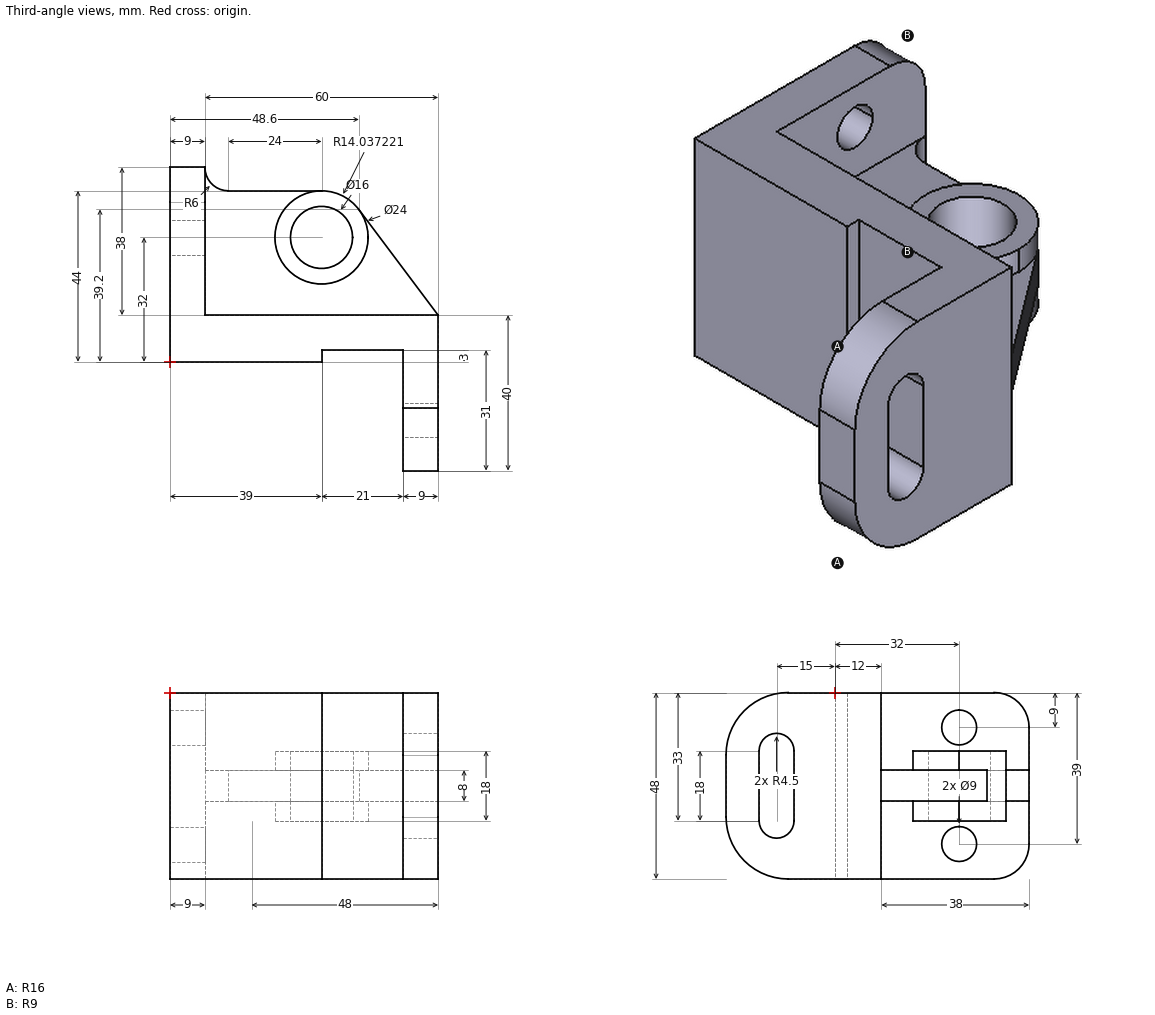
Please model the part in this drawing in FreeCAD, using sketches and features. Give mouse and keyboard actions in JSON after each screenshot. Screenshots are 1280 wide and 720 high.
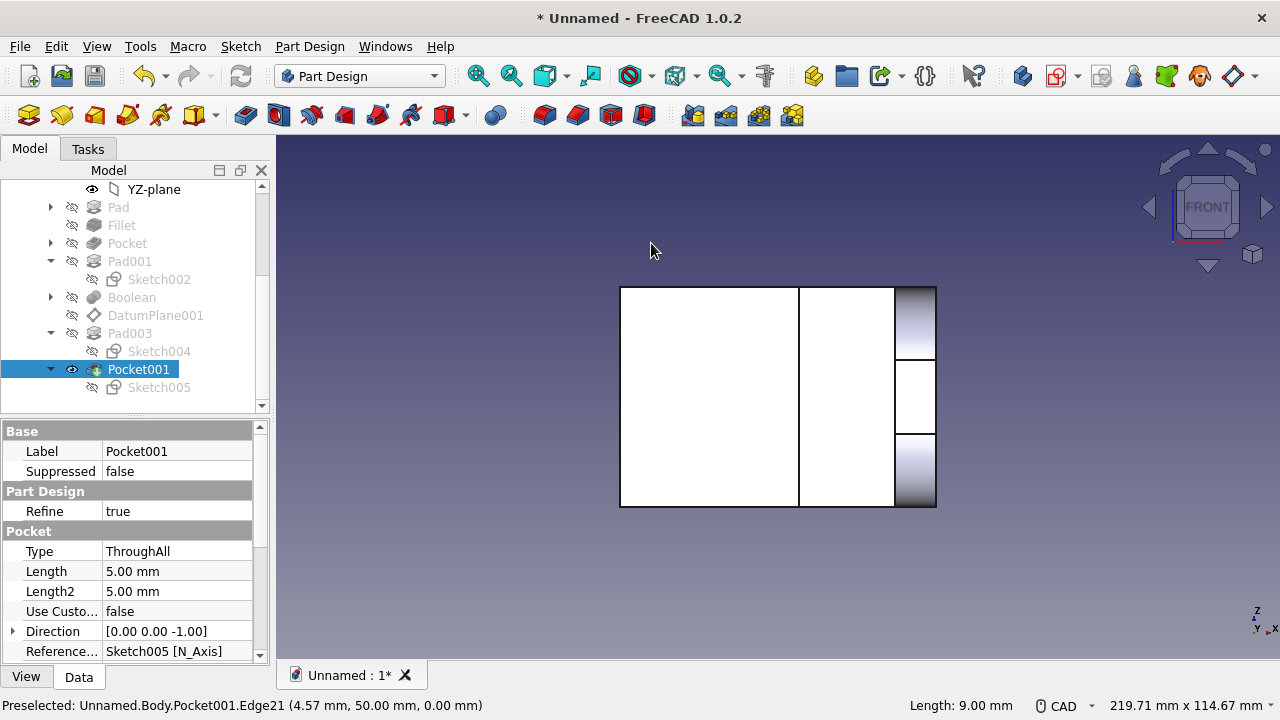
{"action": "key", "text": "3"}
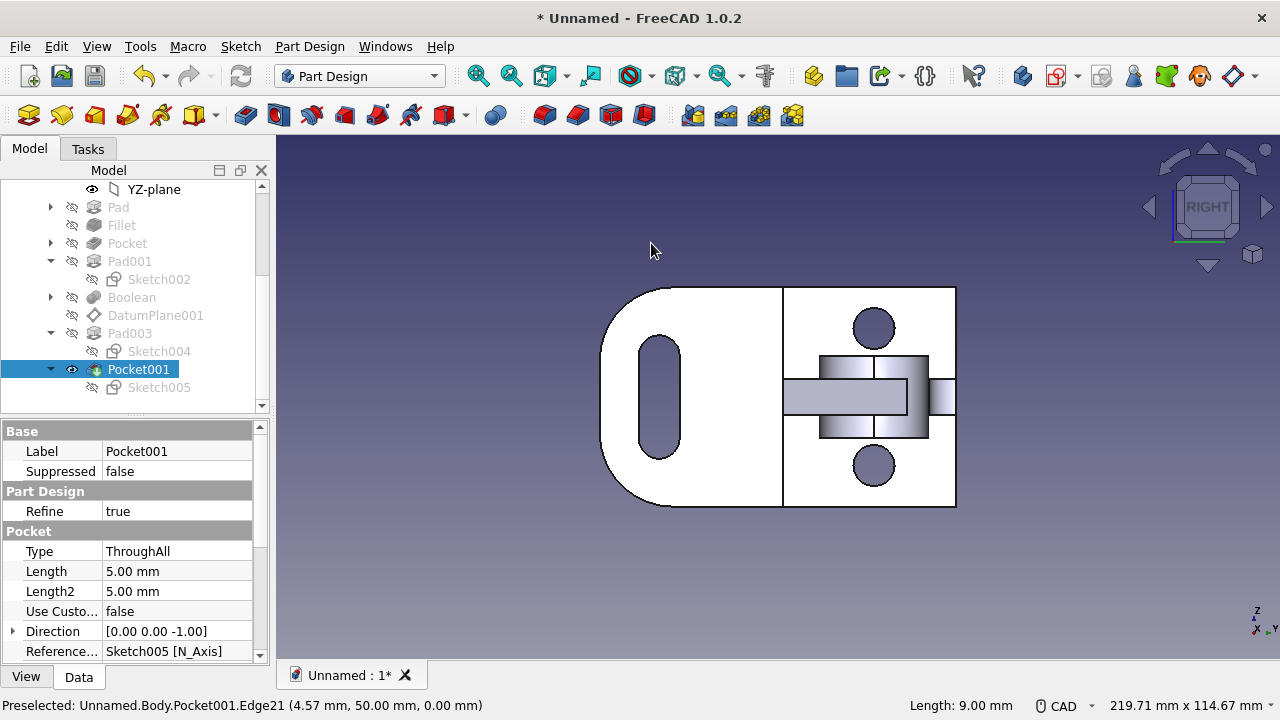
{"action": "key", "text": "v f"}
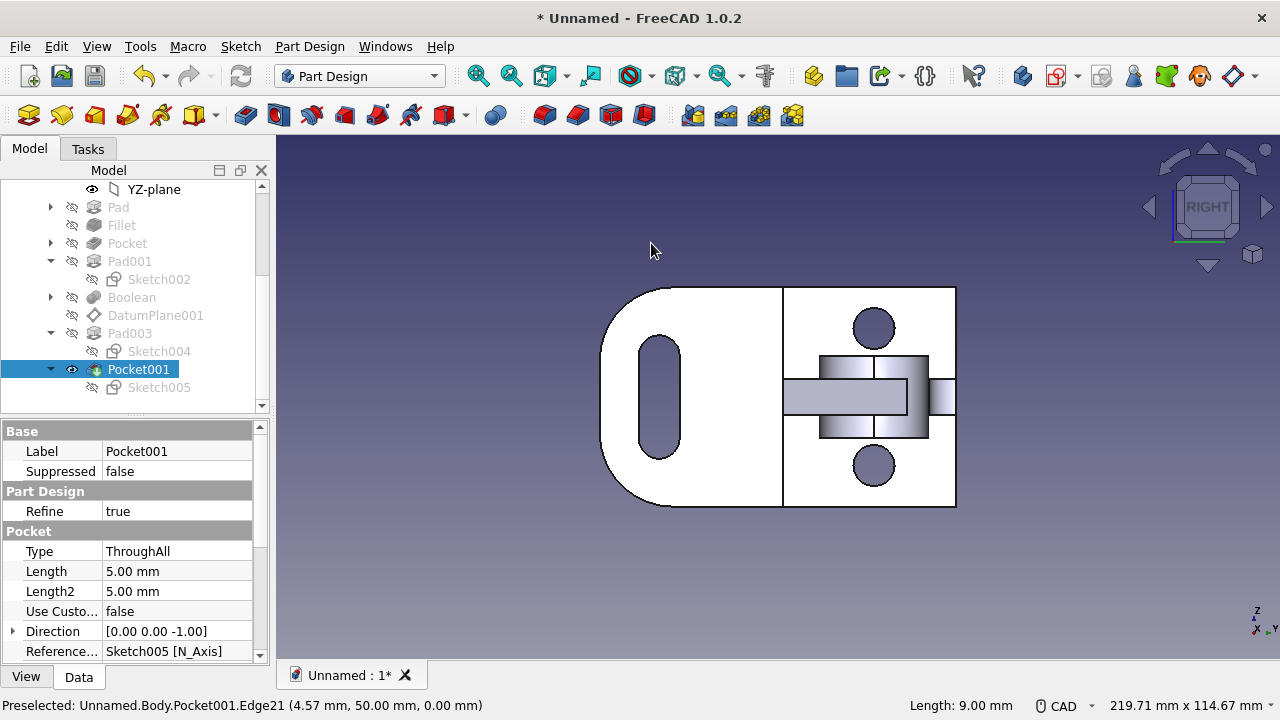
{"action": "key", "text": "5"}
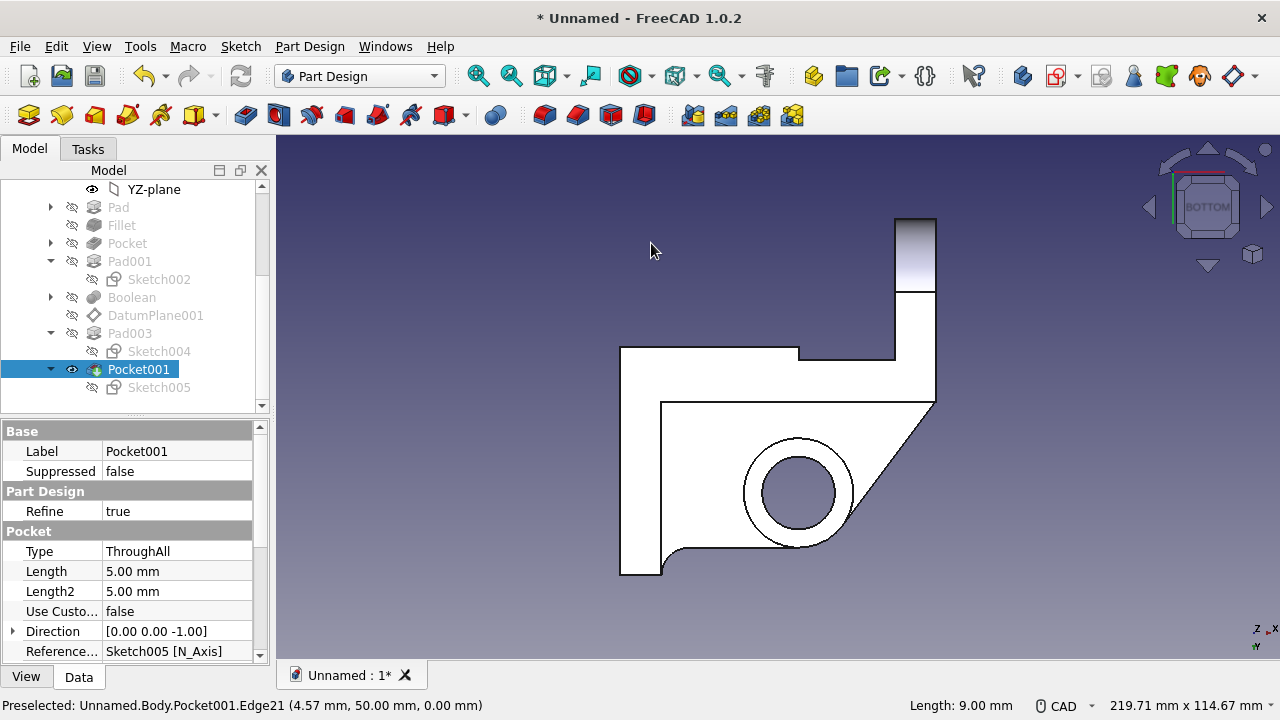
{"action": "left_click", "coordinate": [641, 574], "text": "ctrl"}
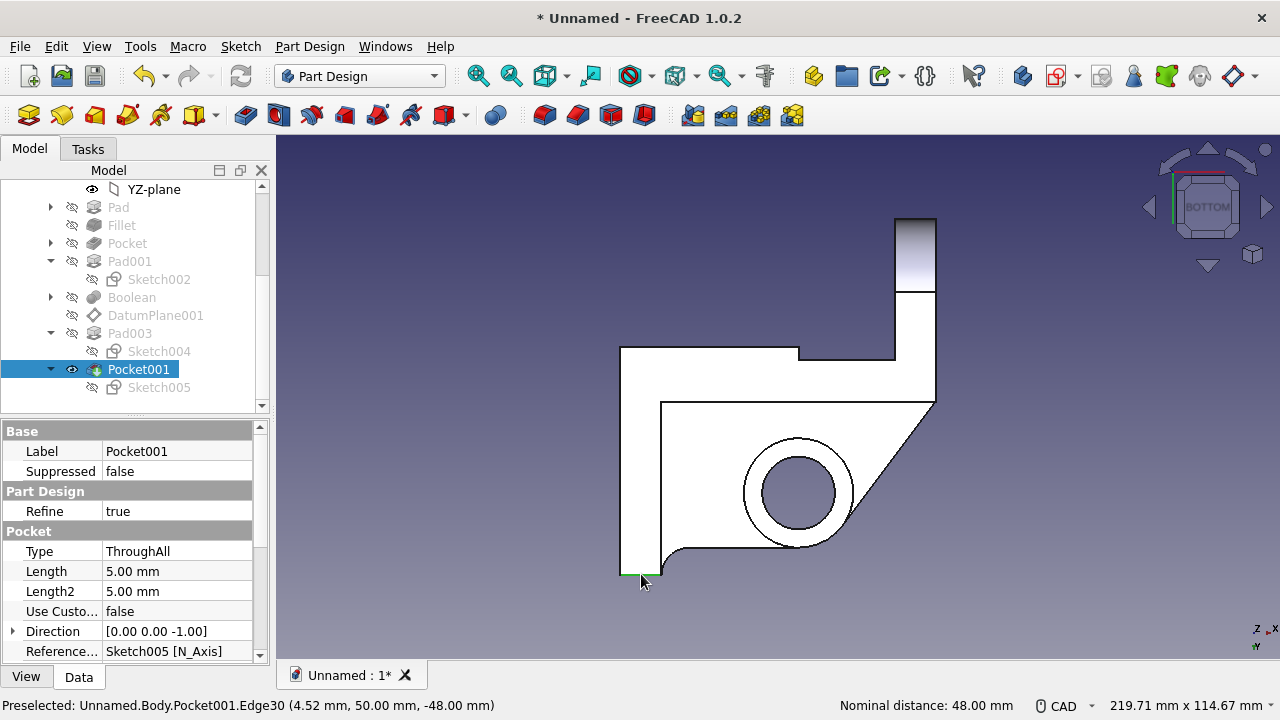
{"action": "left_click", "coordinate": [545, 116]}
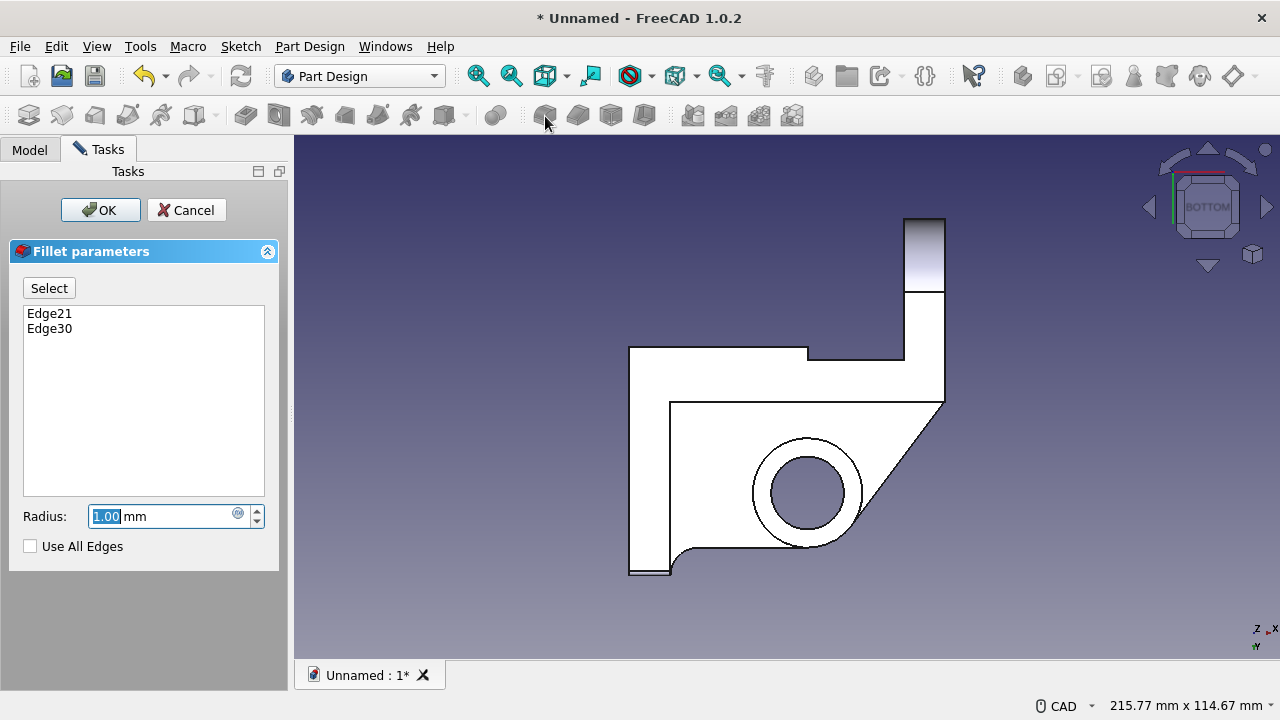
{"action": "type", "text": "9"}
{"action": "key", "text": "Tab"}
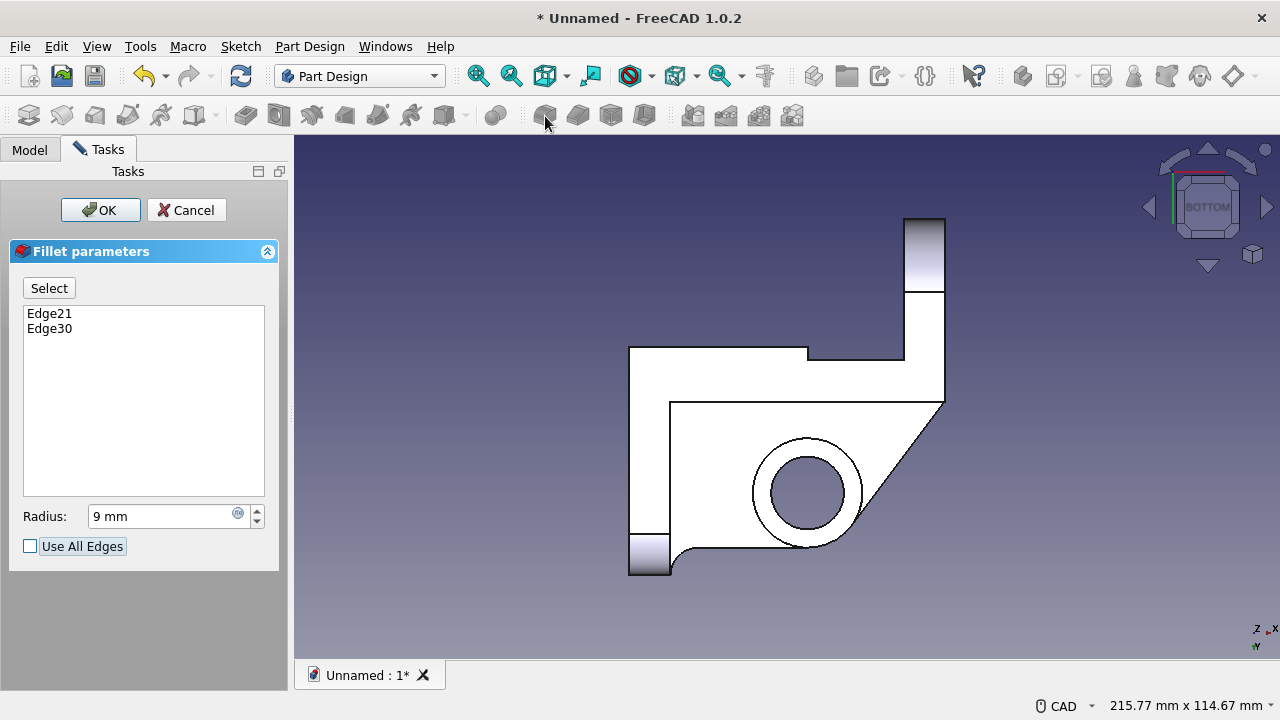
{"action": "left_click", "coordinate": [101, 210]}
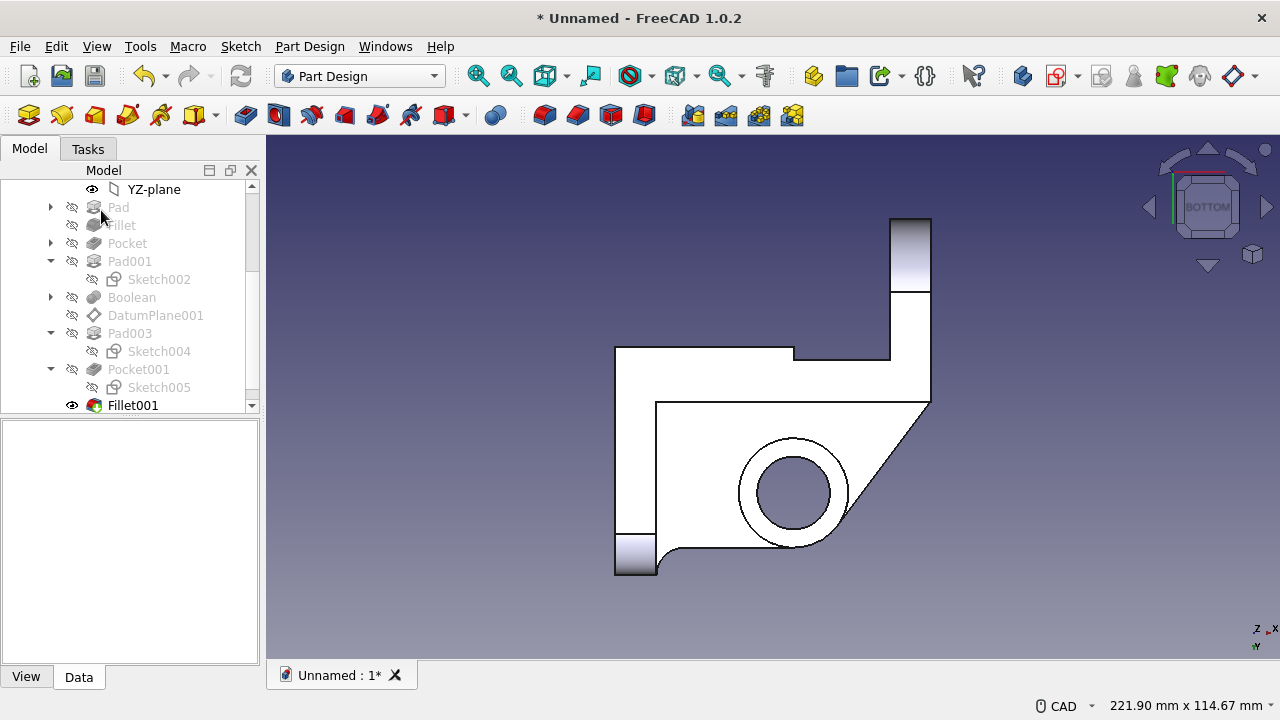
{"action": "key", "text": "0"}